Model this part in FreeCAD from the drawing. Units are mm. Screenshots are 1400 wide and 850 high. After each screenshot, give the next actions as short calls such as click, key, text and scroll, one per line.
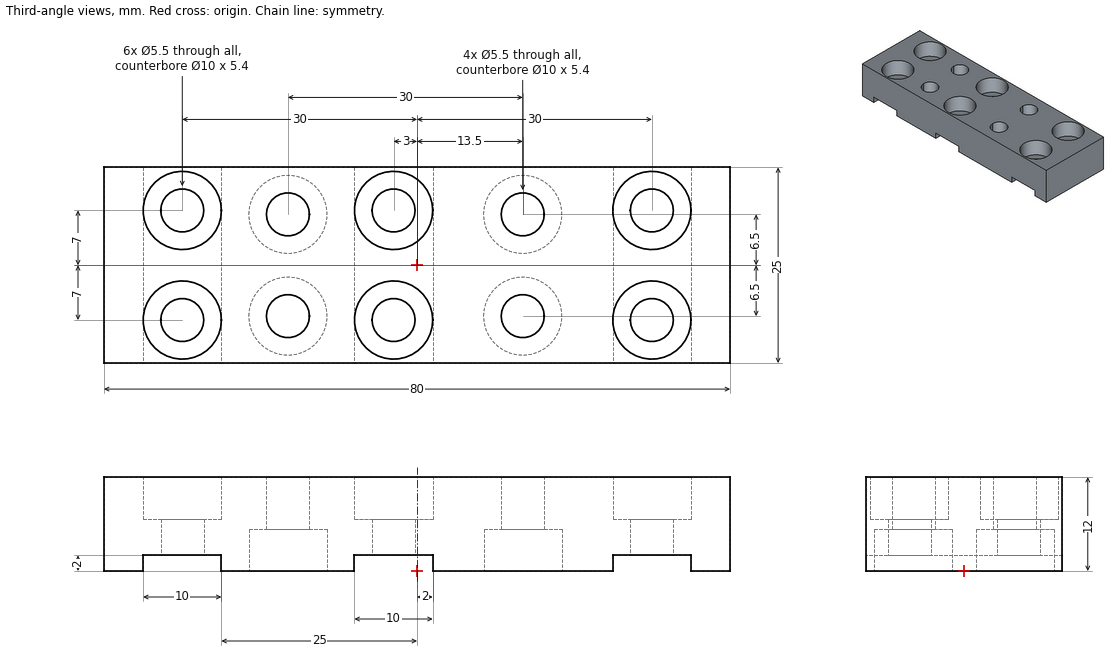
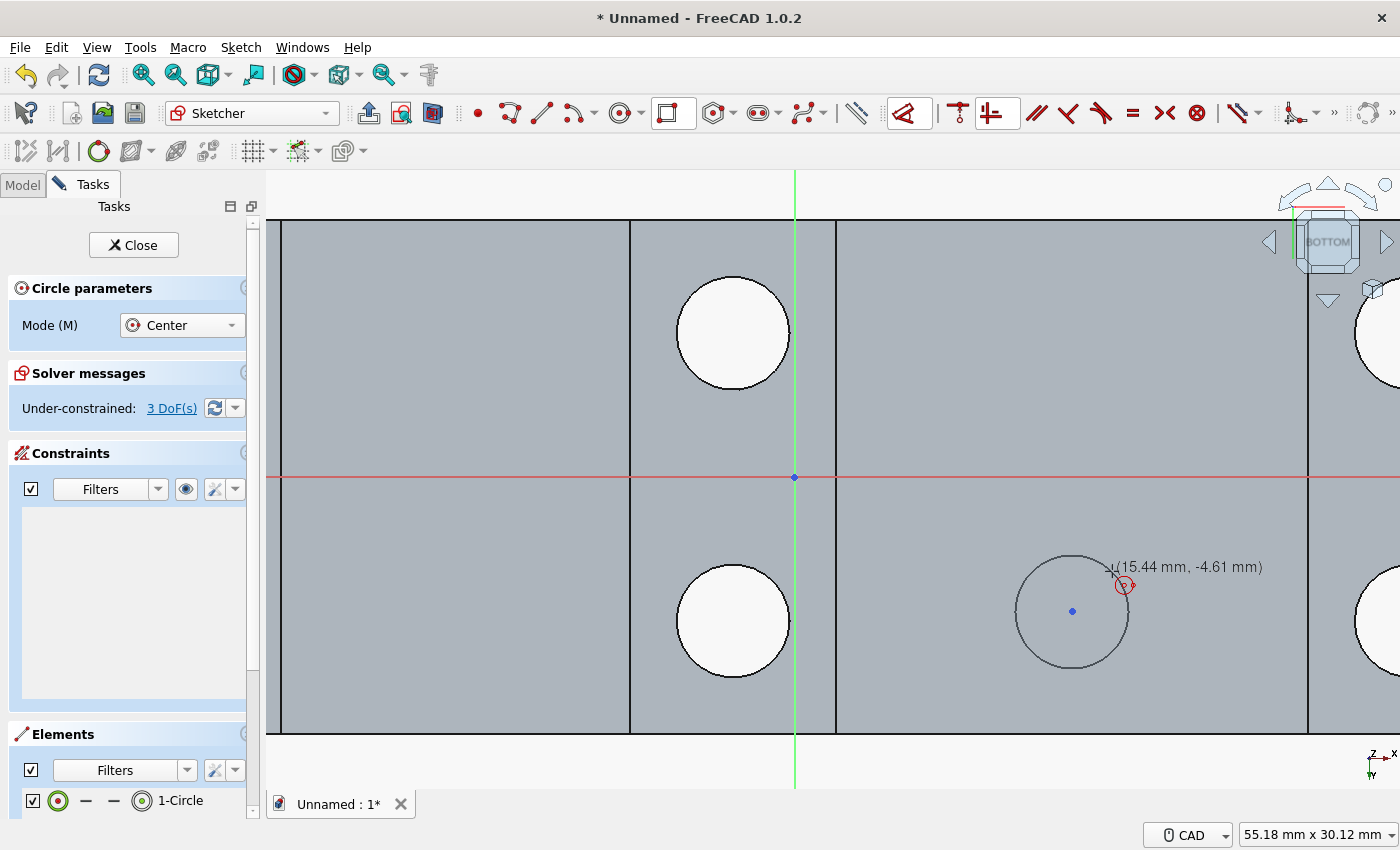
click(1072, 344)
click(1112, 304)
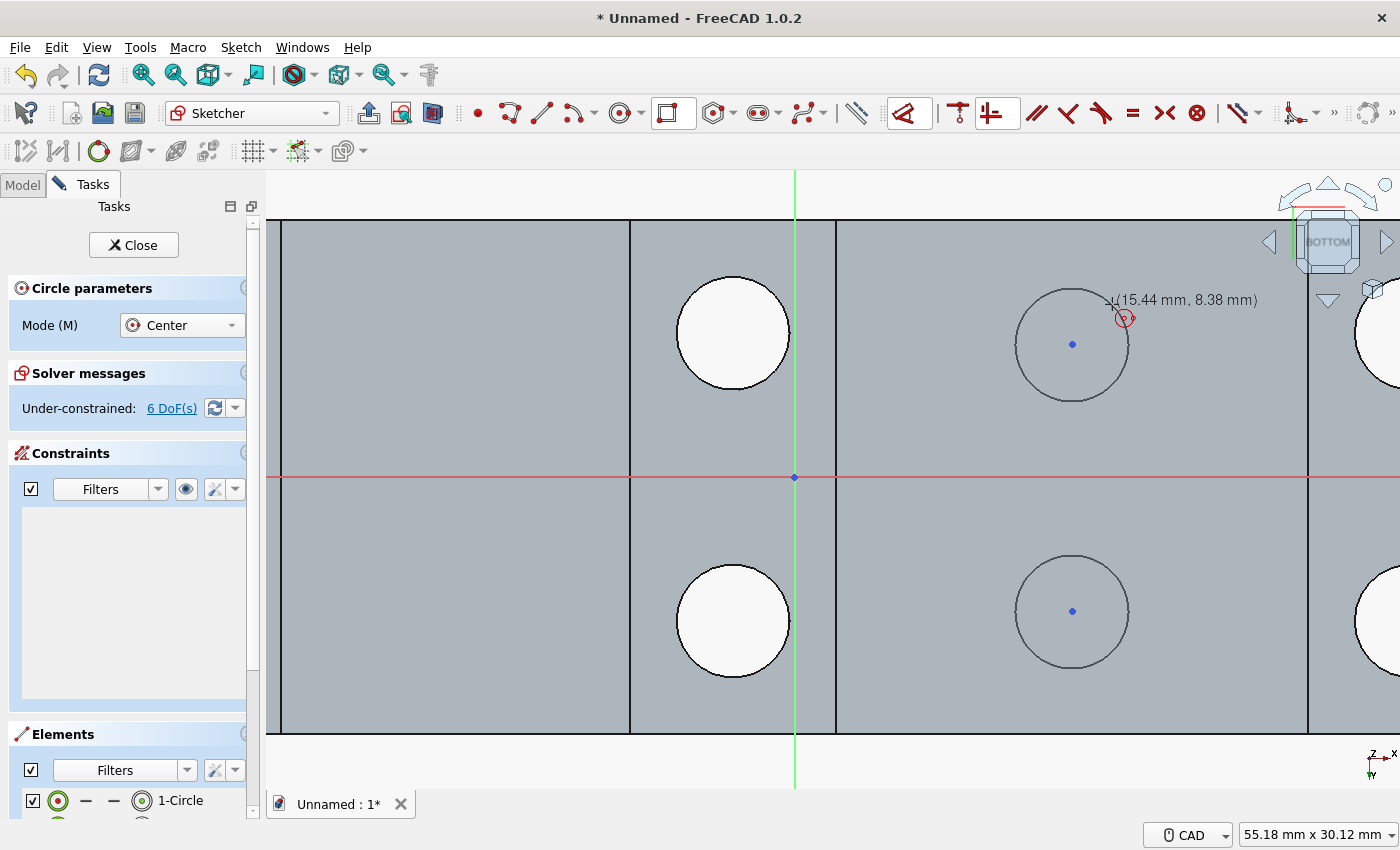
click(456, 611)
click(496, 571)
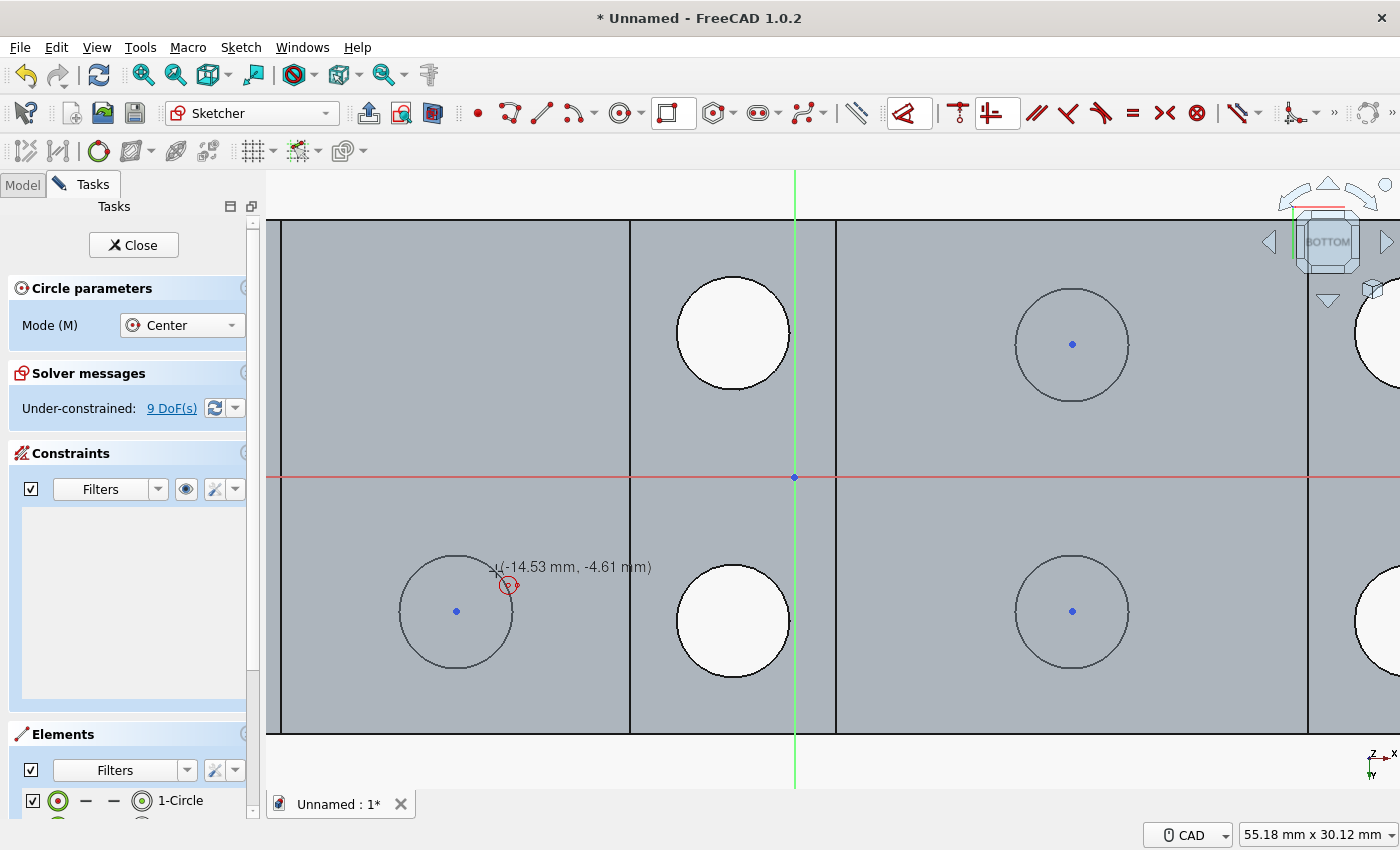
click(456, 344)
click(496, 304)
key(Escape)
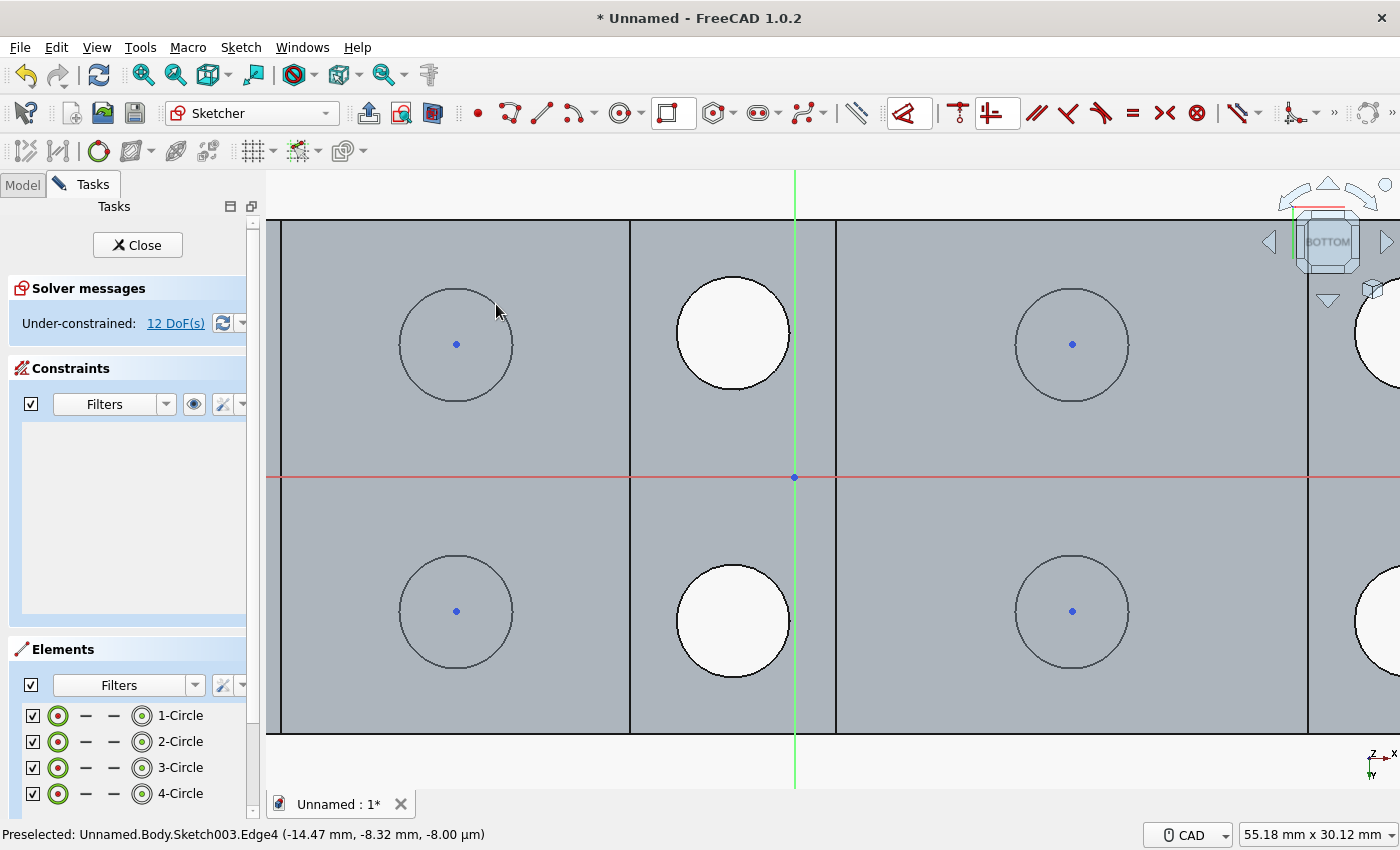
click(1112, 572)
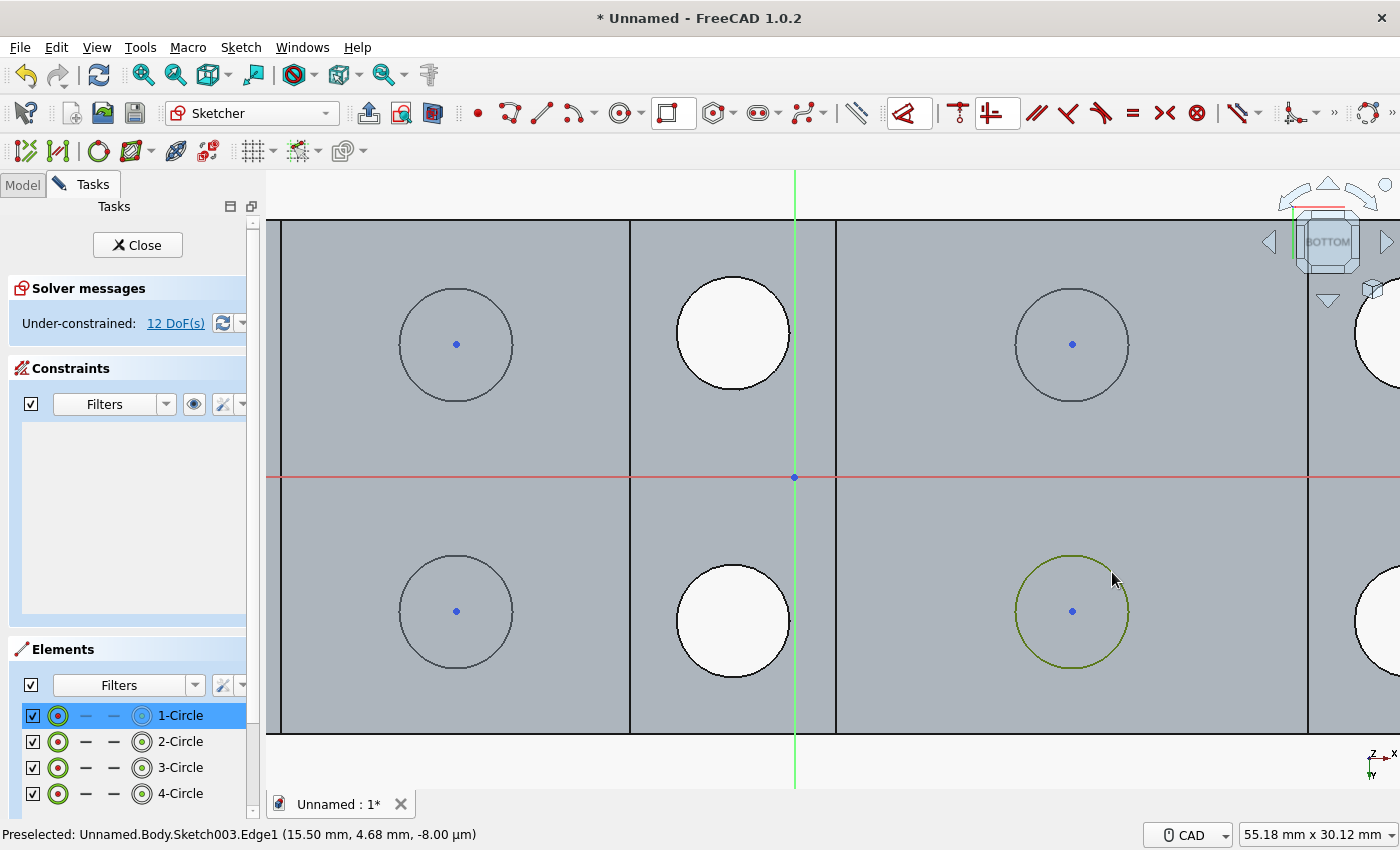
click(1112, 305)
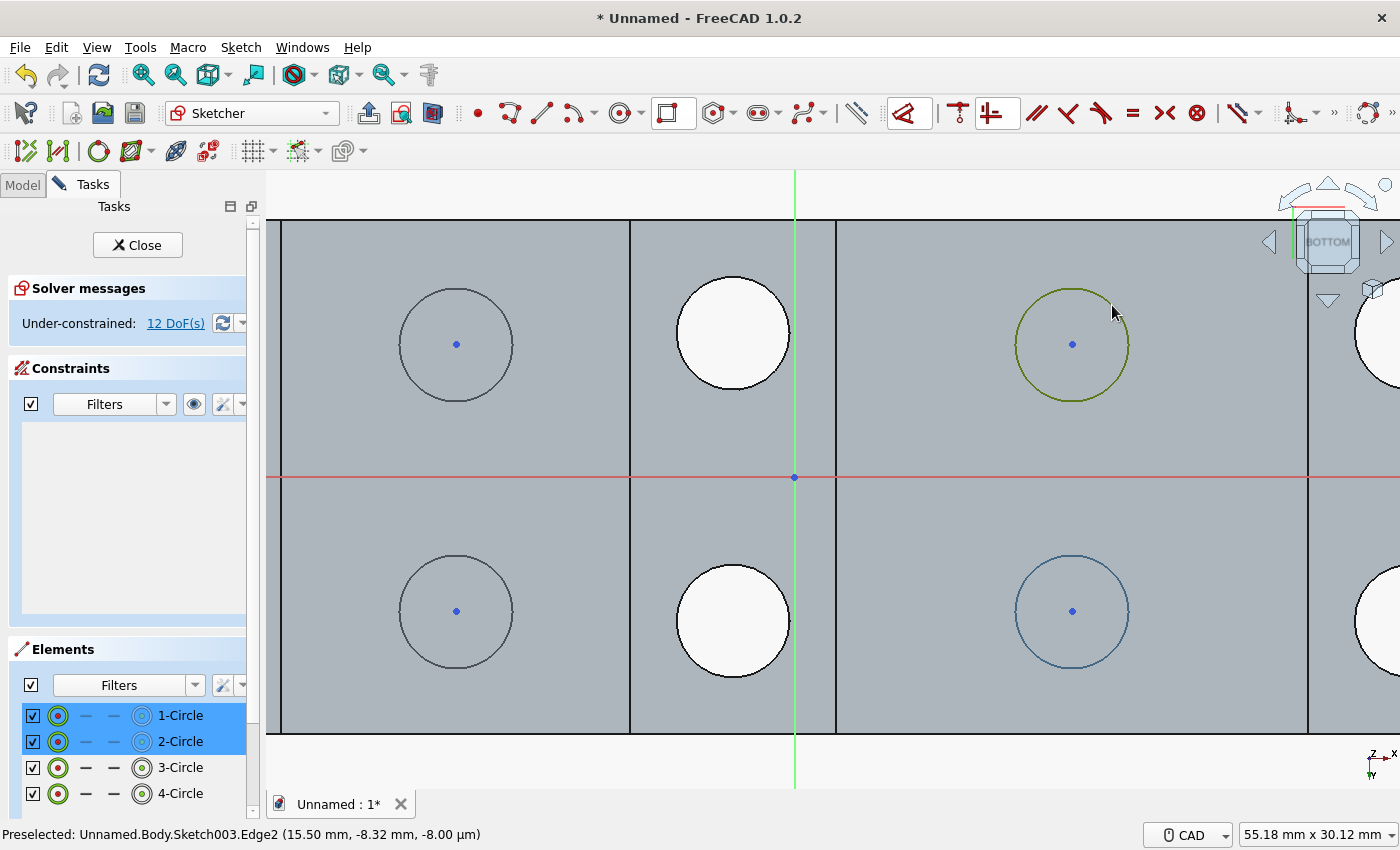
click(496, 572)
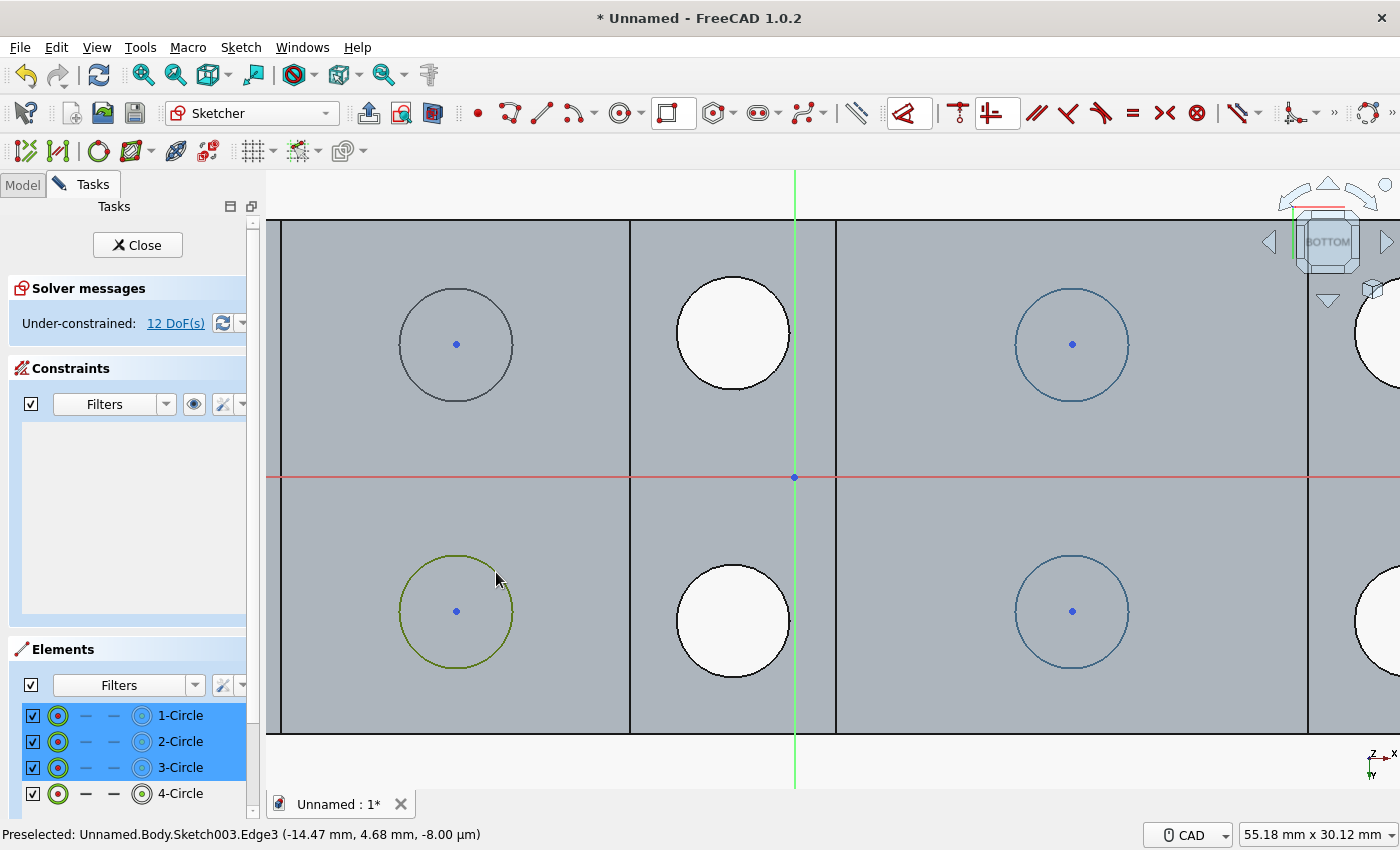
click(496, 305)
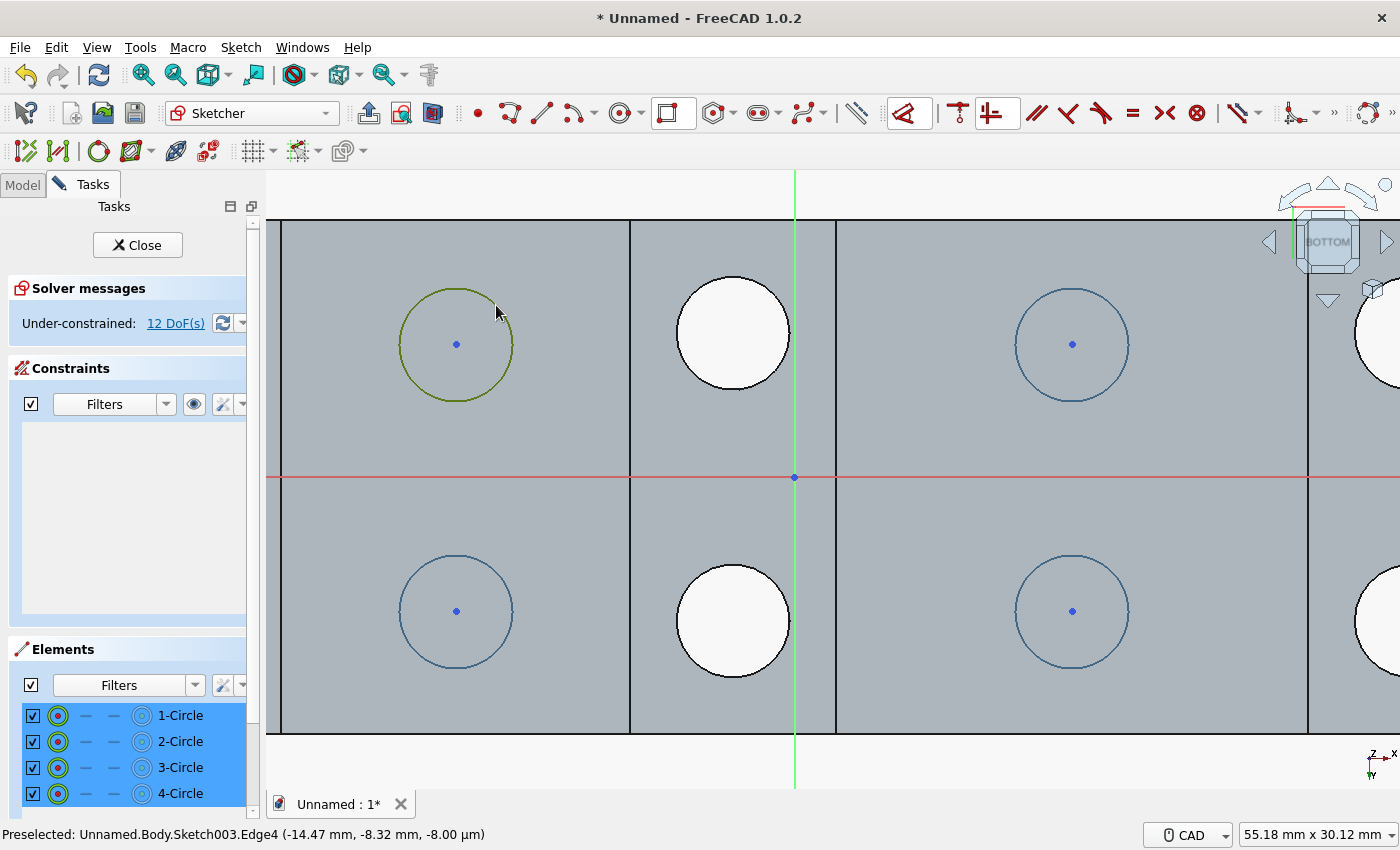
click(1134, 114)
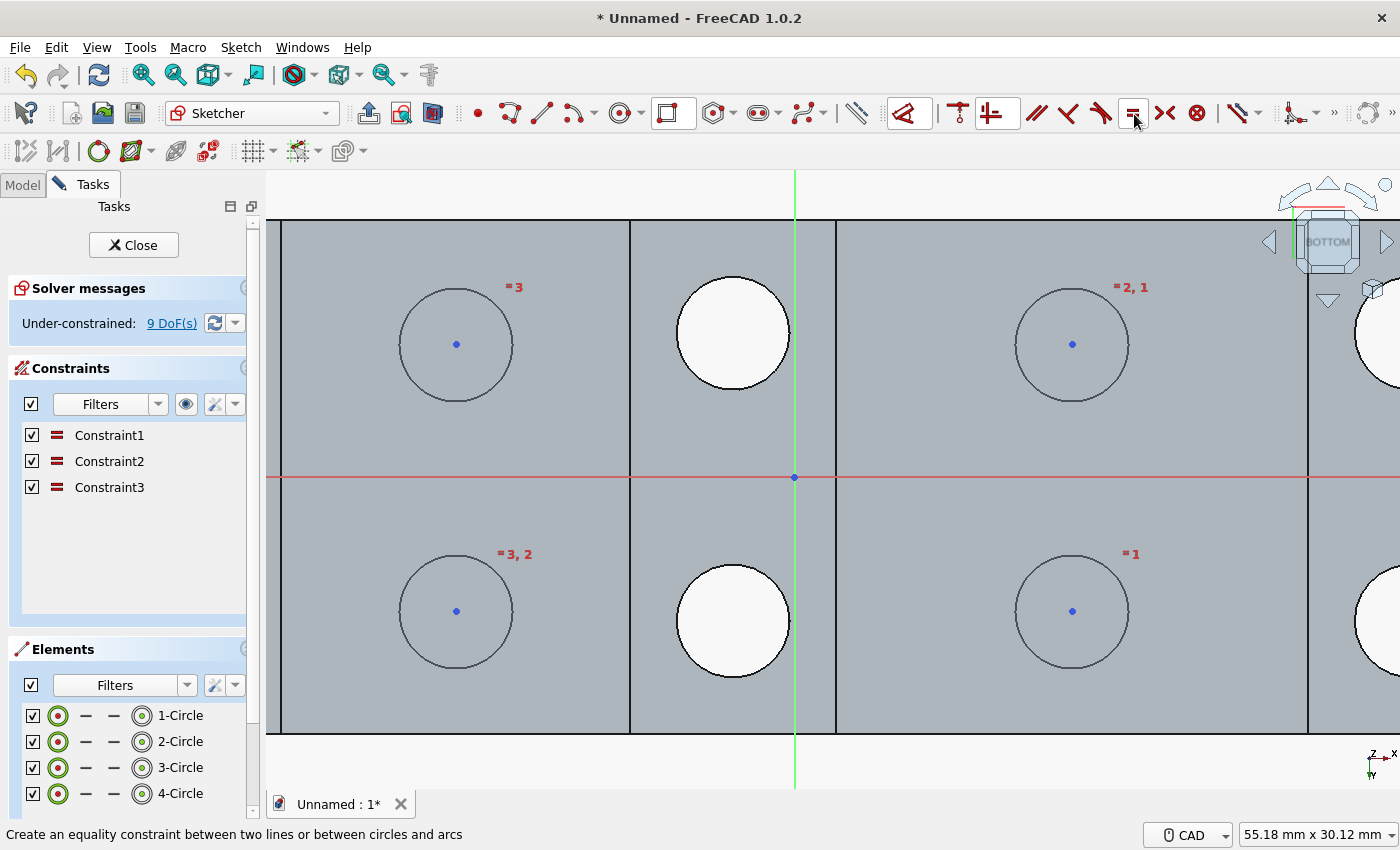
click(1072, 612)